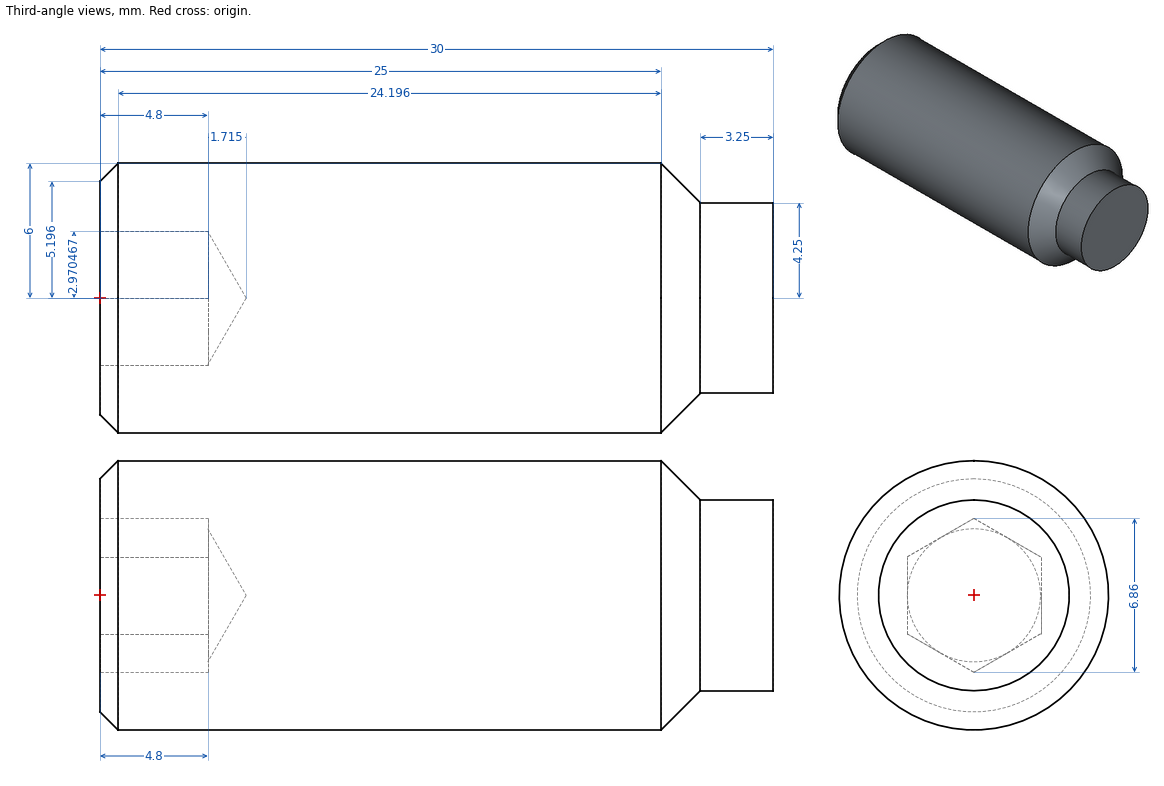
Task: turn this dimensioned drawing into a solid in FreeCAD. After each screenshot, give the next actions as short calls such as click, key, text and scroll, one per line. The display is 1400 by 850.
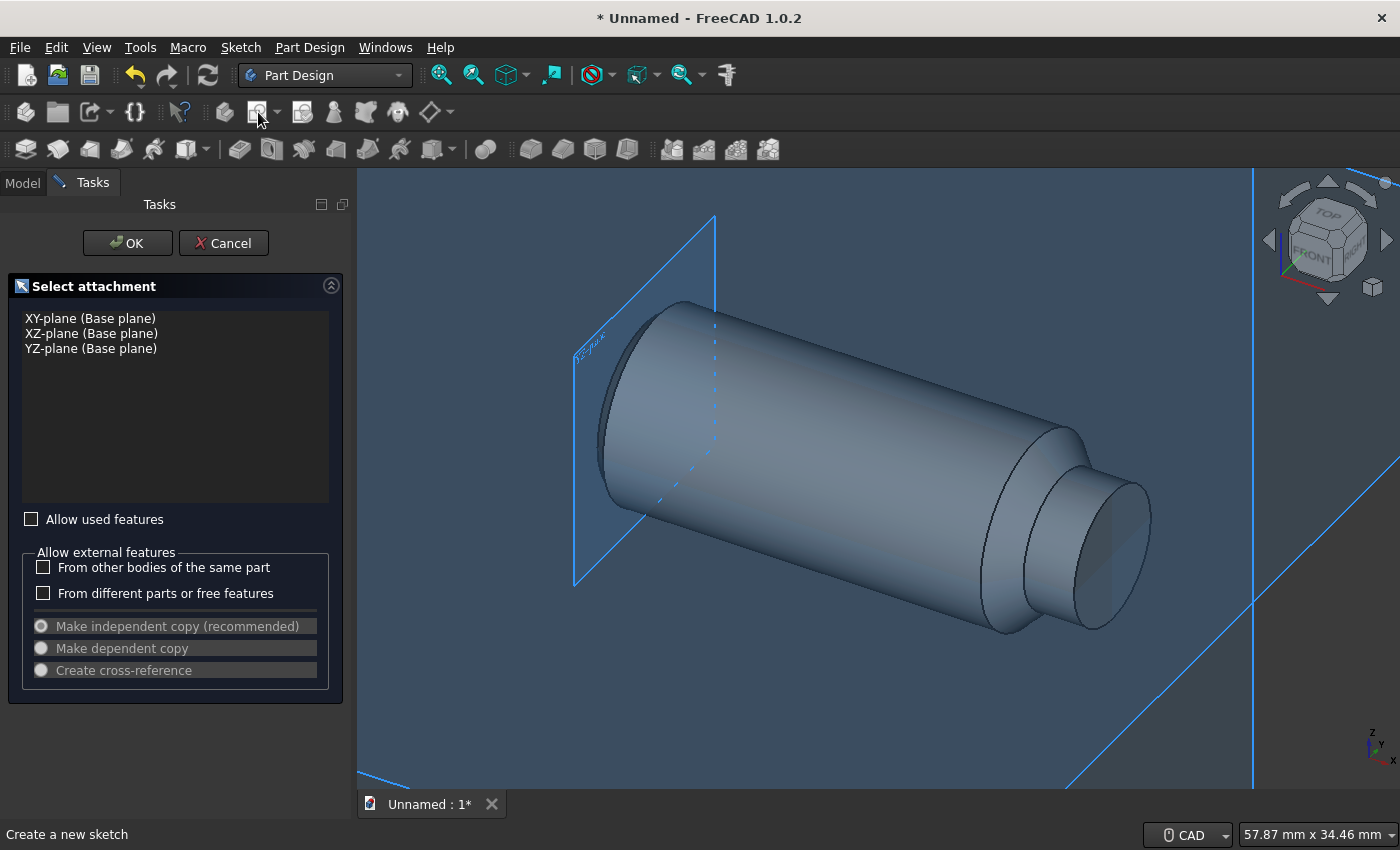
click(82, 348)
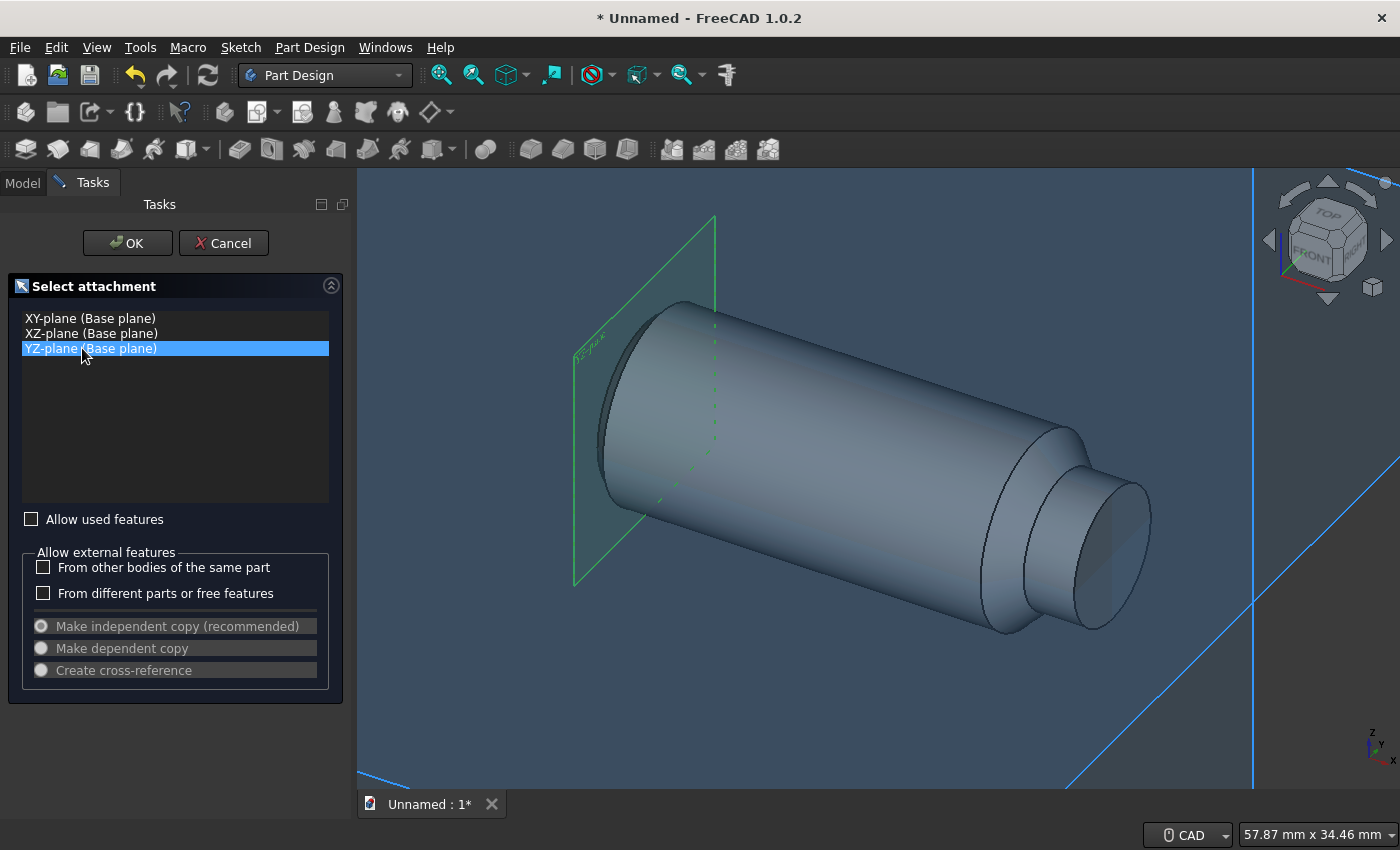
click(128, 243)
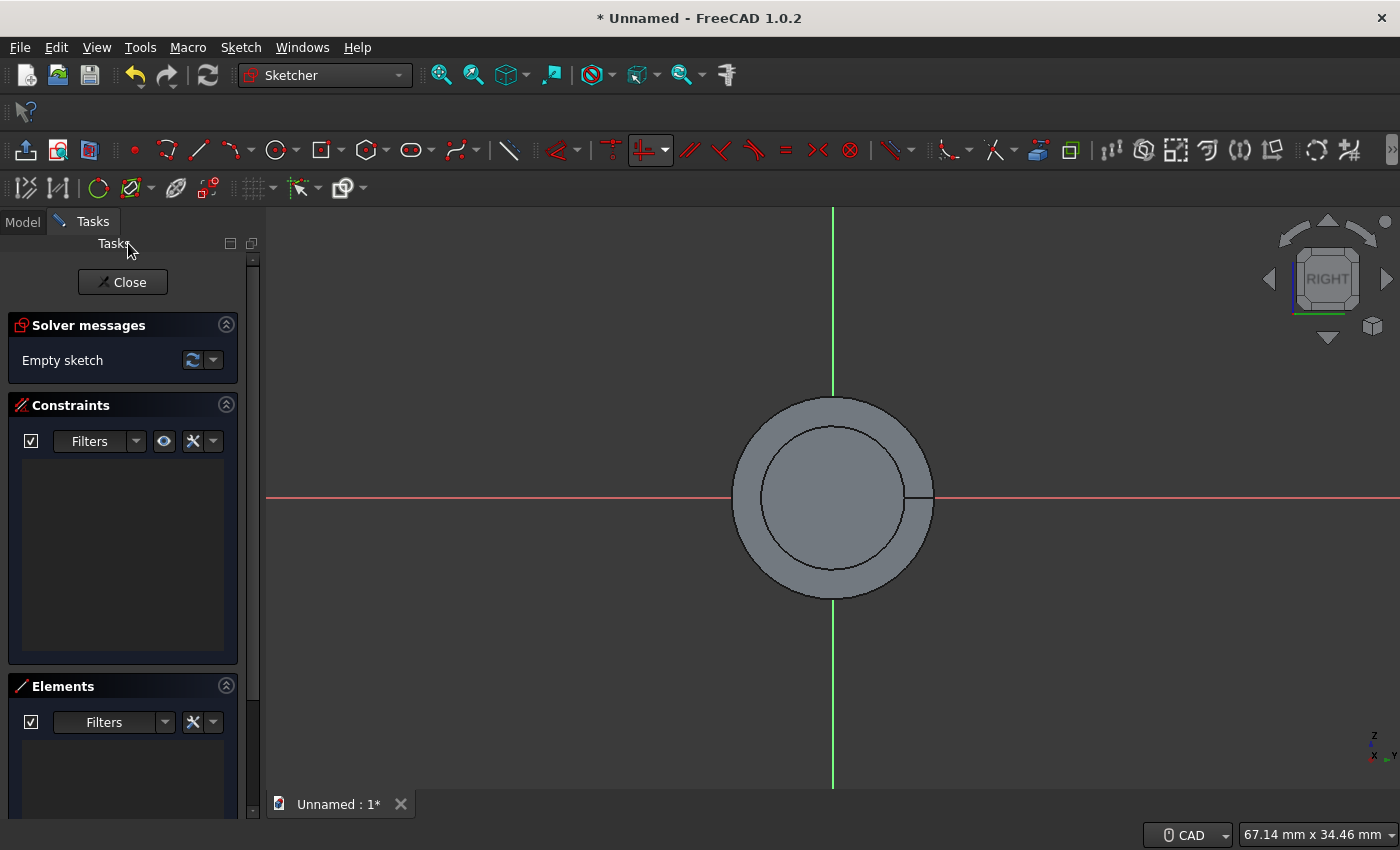
click(90, 150)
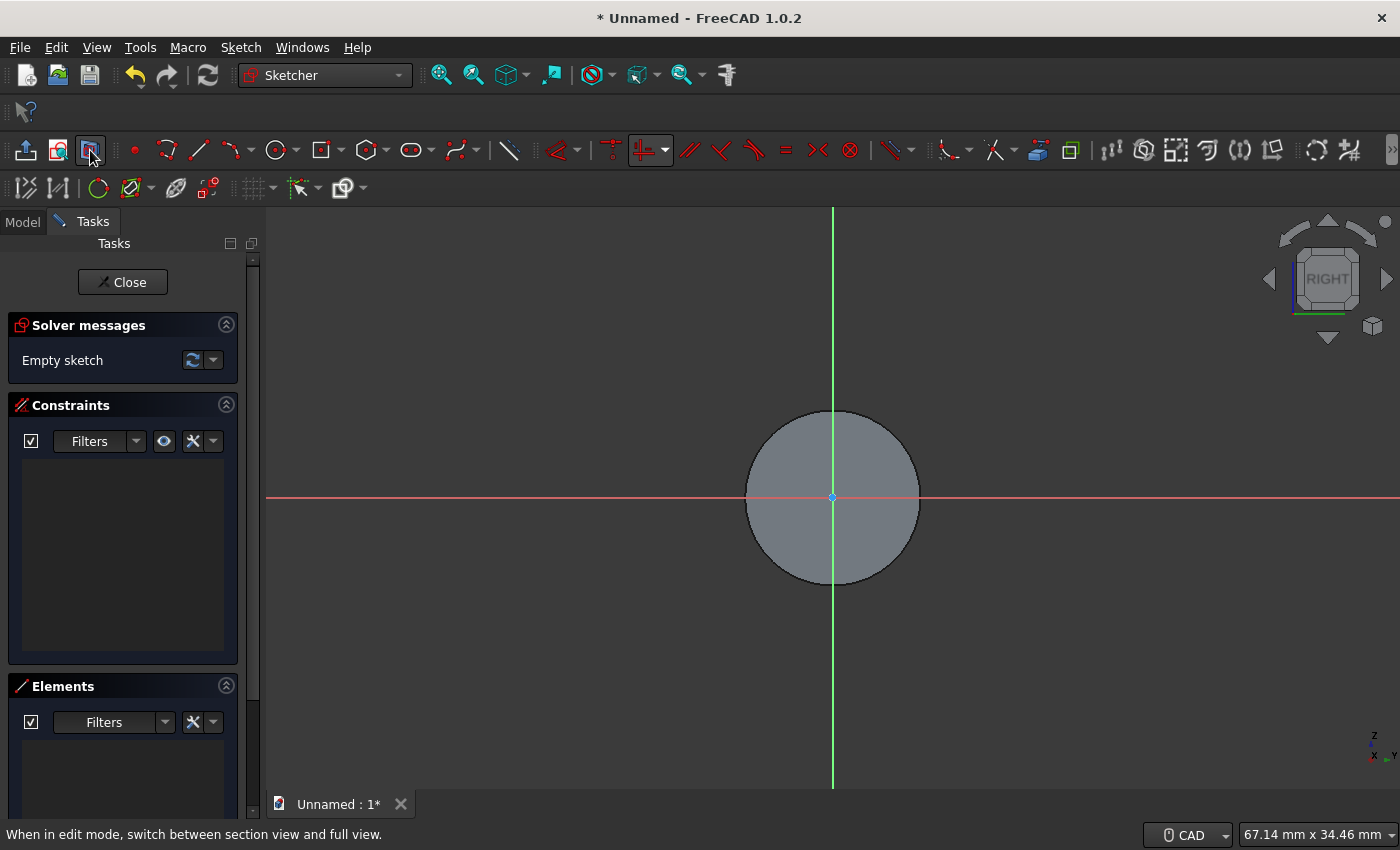
scroll(862, 498, up, 6)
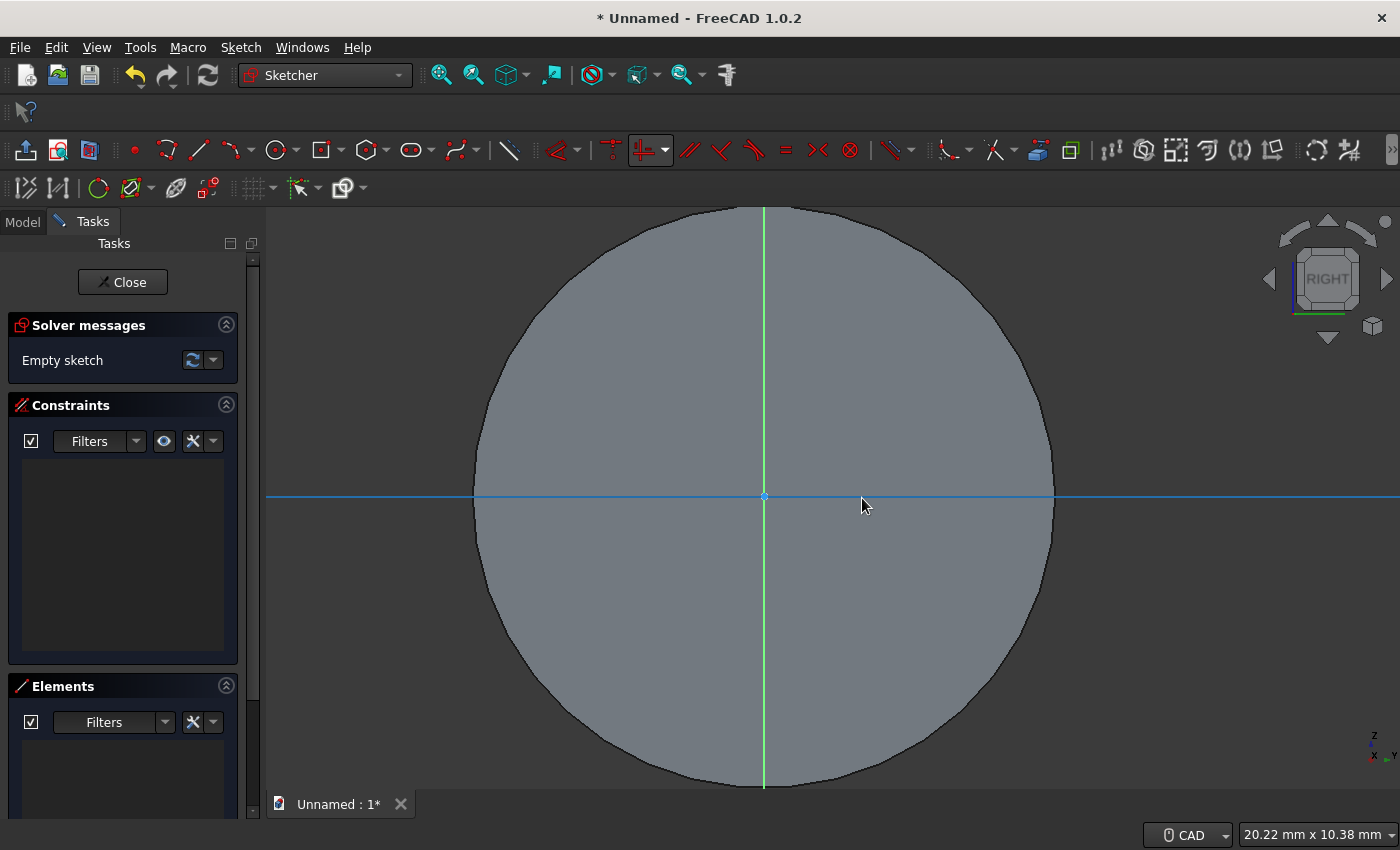
click(366, 150)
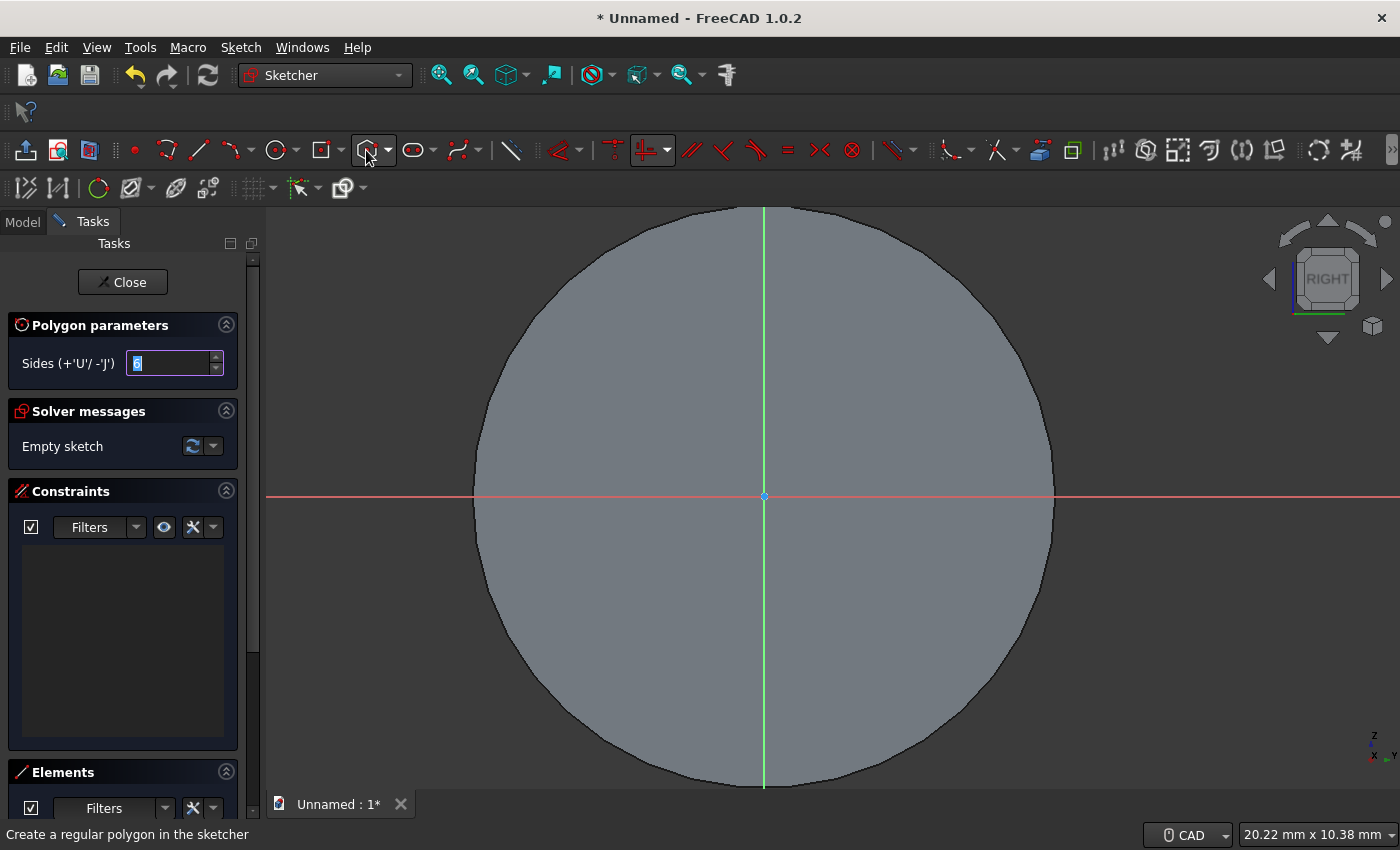
click(764, 497)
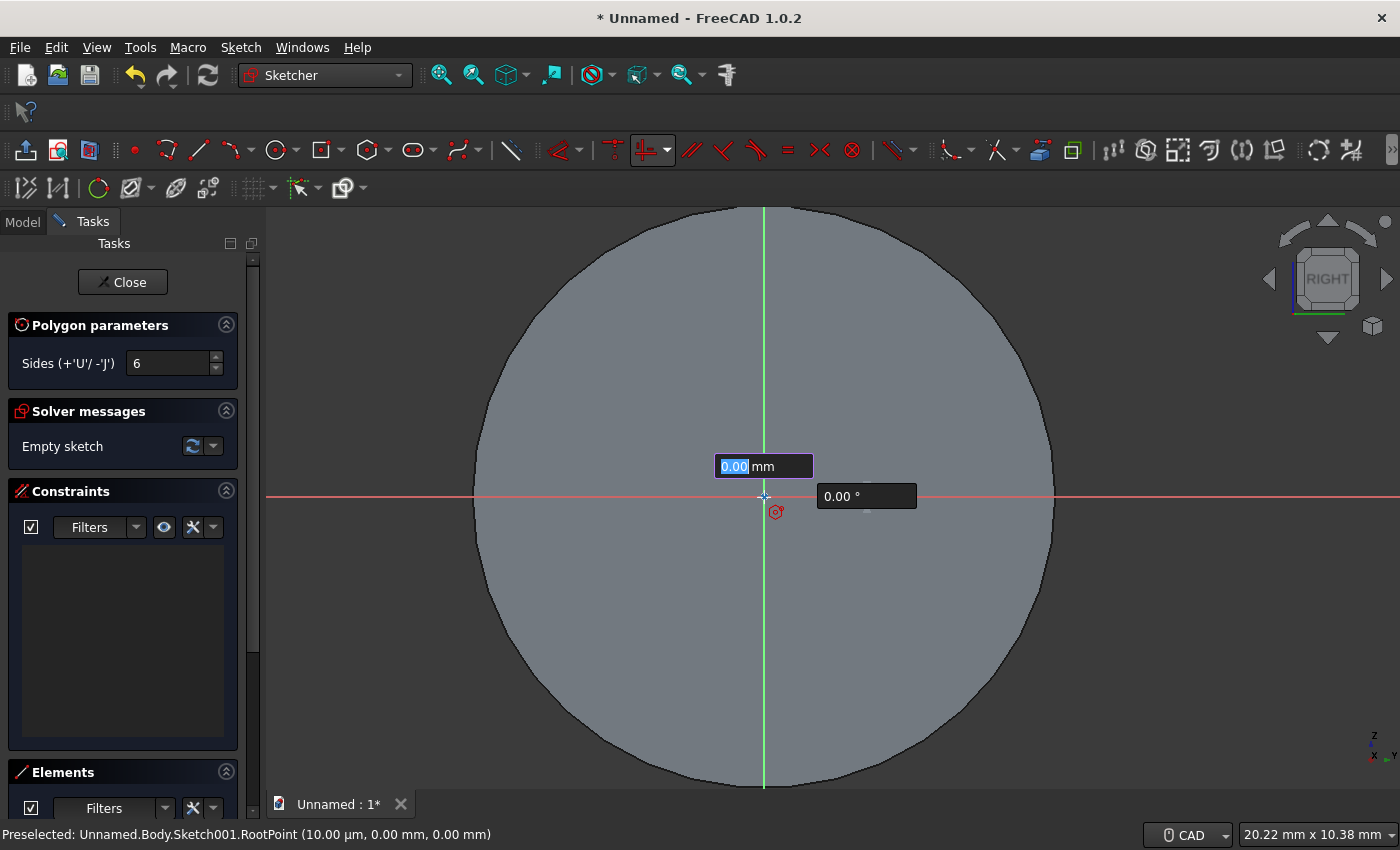
click(764, 304)
right_click(764, 304)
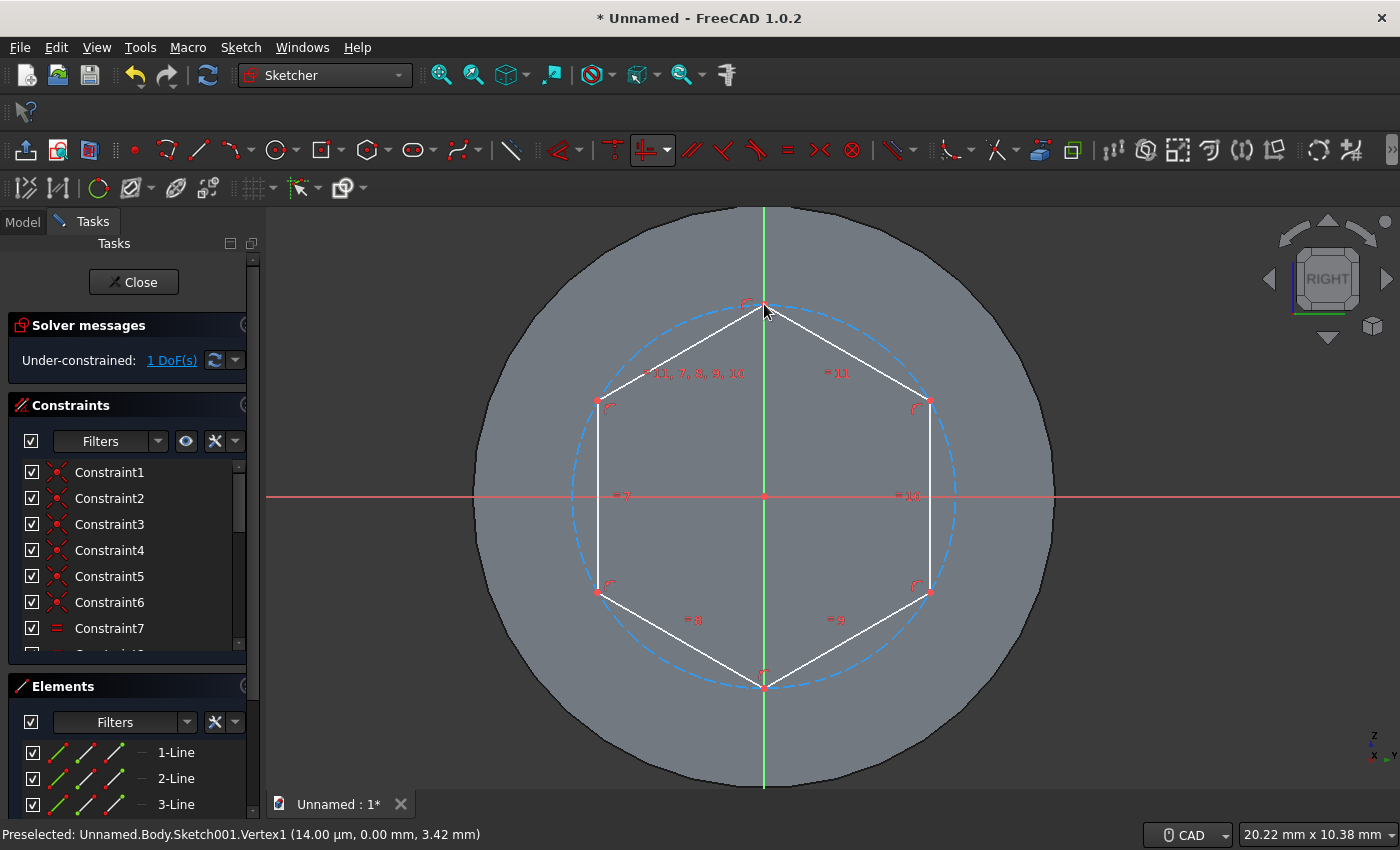
key(d)